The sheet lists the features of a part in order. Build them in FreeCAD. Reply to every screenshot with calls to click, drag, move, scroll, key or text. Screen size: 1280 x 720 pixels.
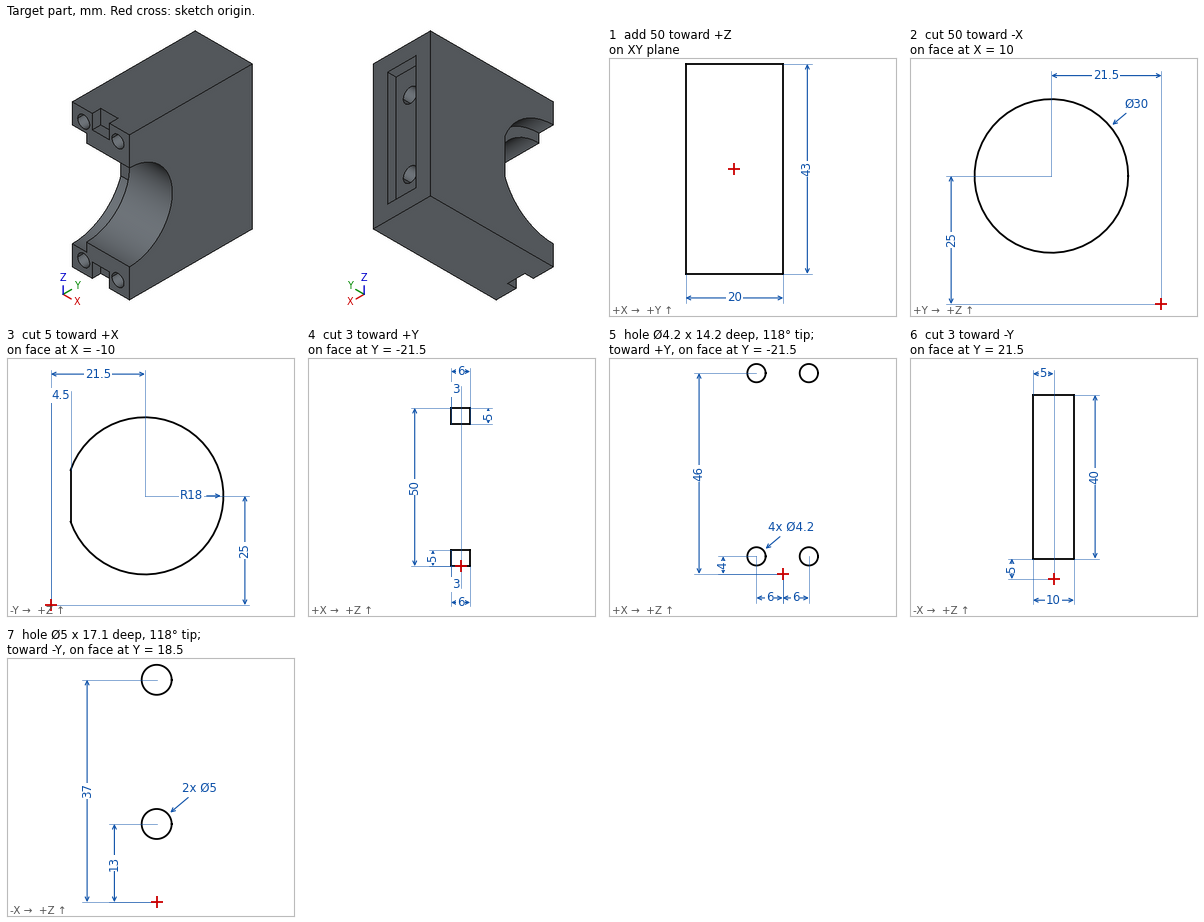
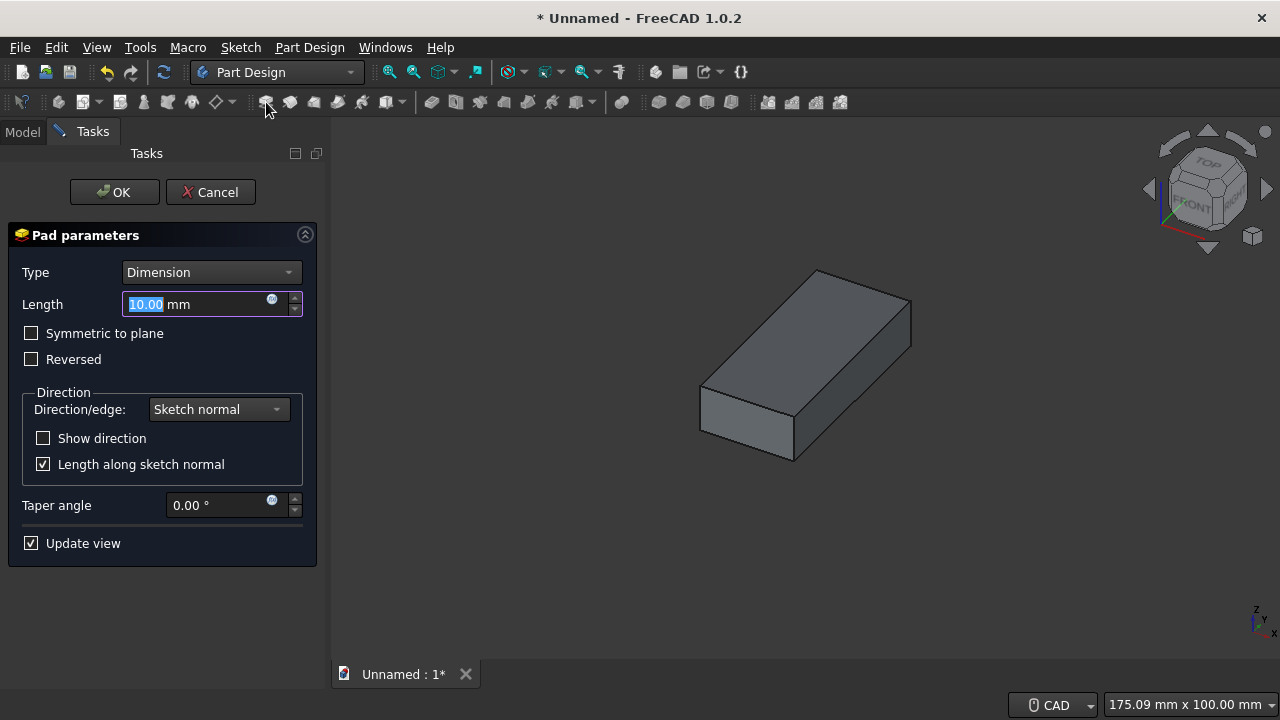
text(50)
key(Tab)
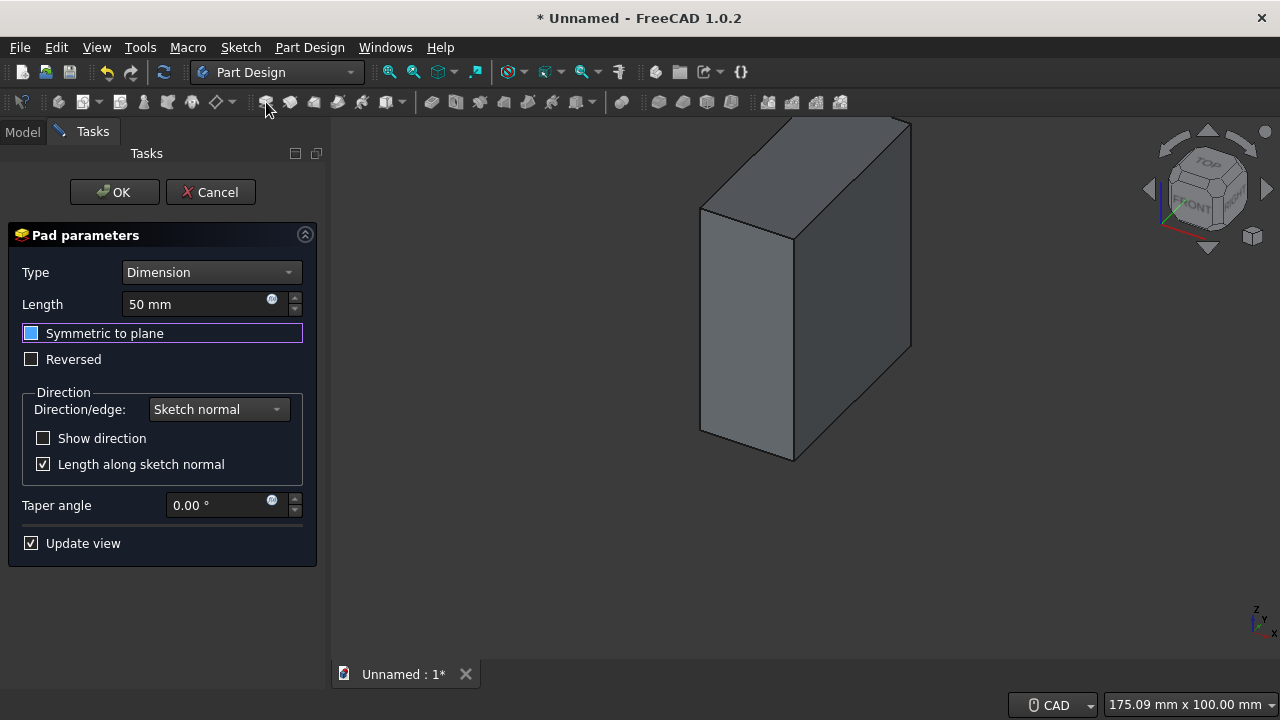
click(115, 192)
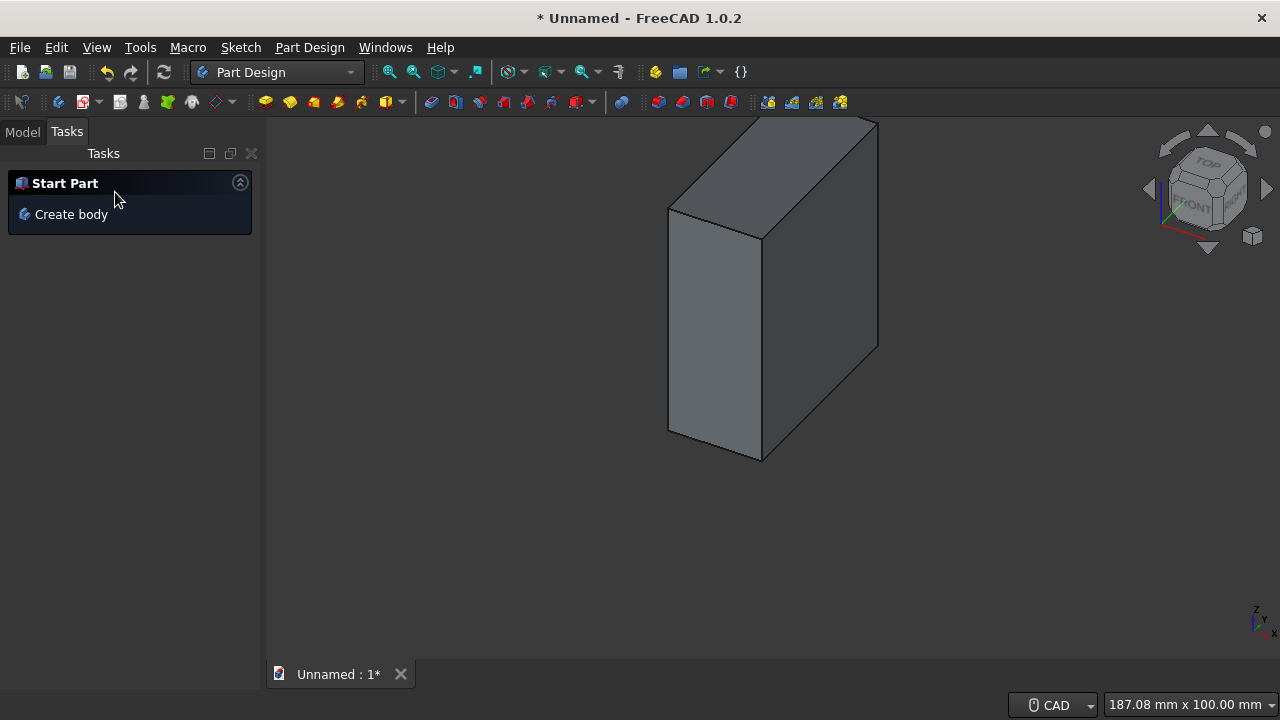
click(390, 72)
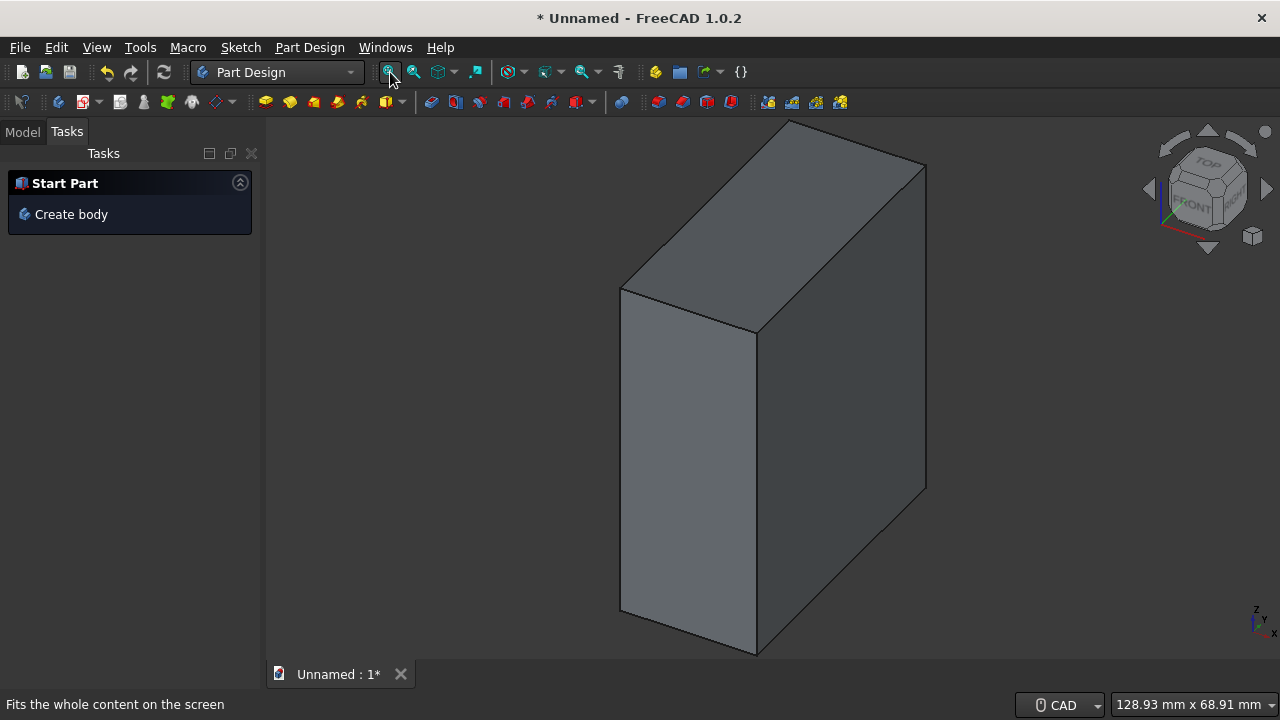
click(841, 410)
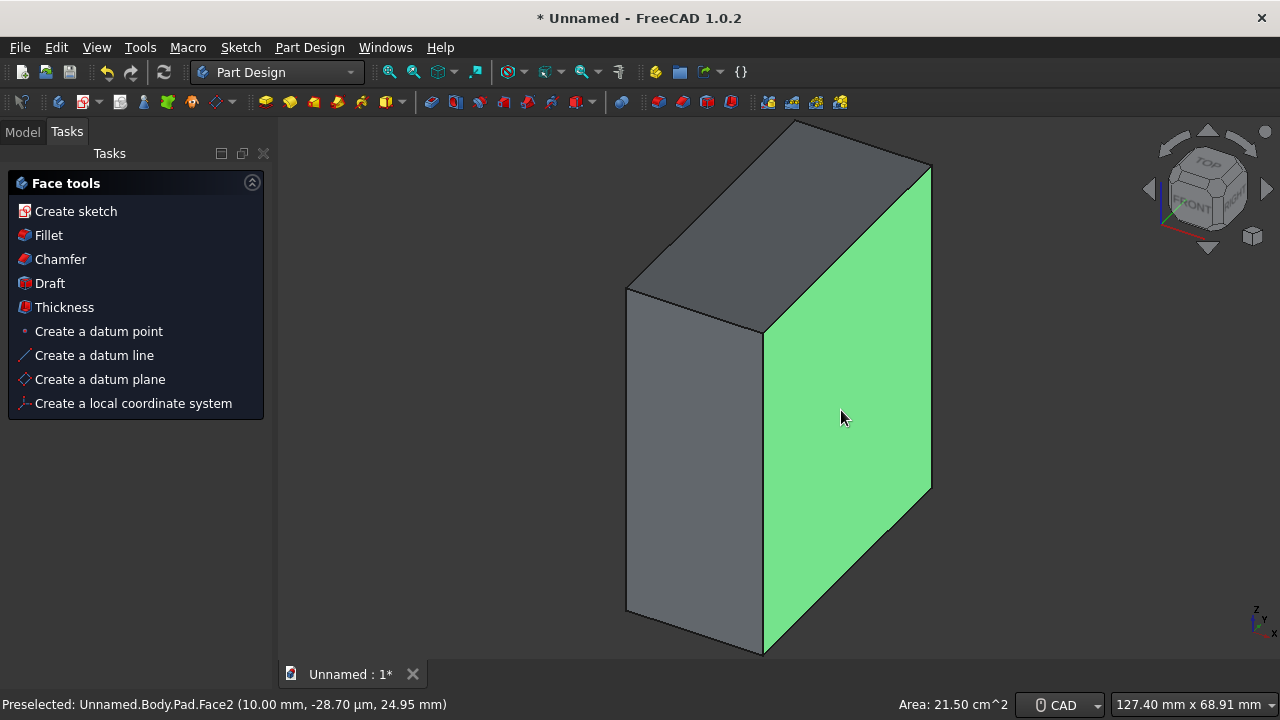
click(84, 102)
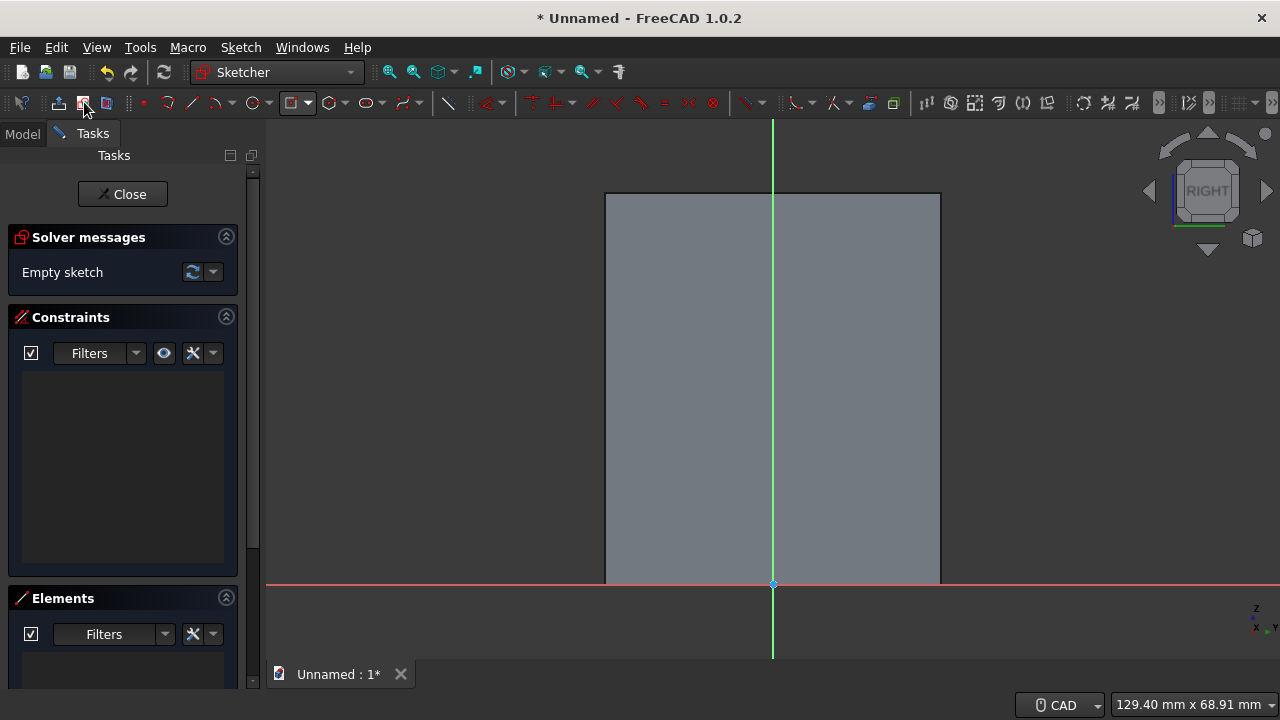
click(254, 104)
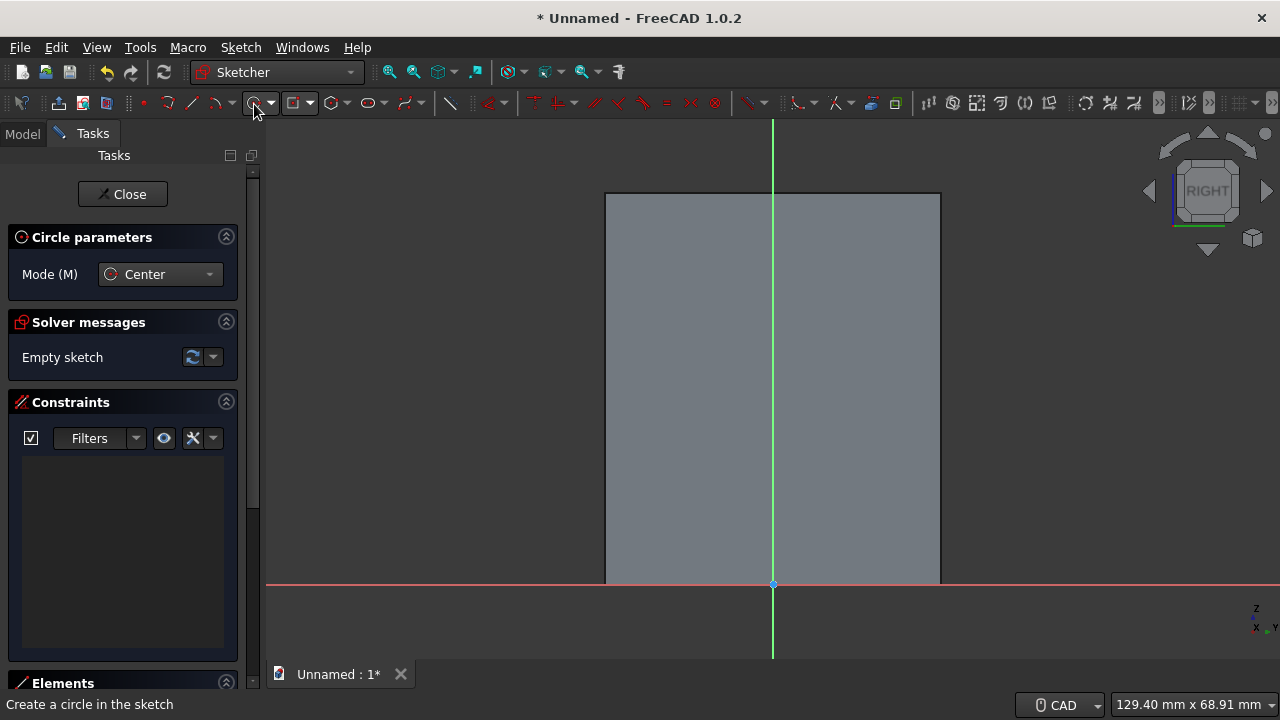
click(605, 389)
move(688, 306)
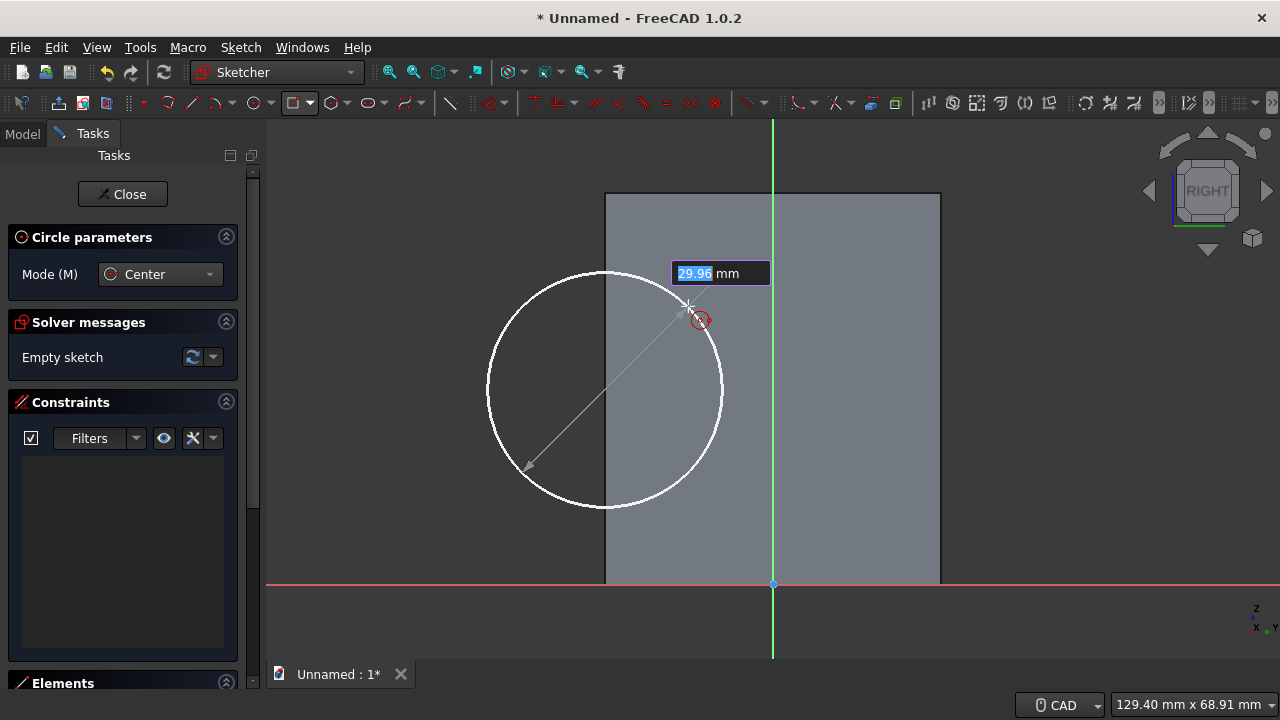
text(30)
key(Return)
key(Escape)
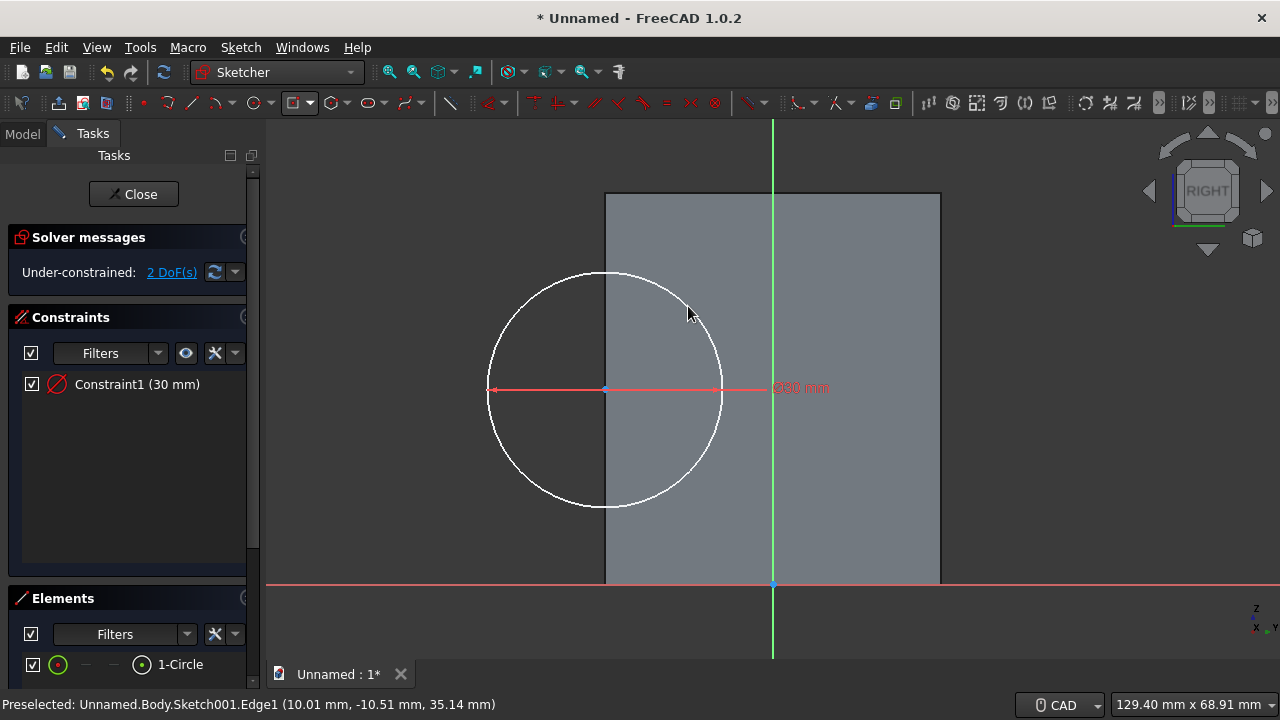
click(488, 104)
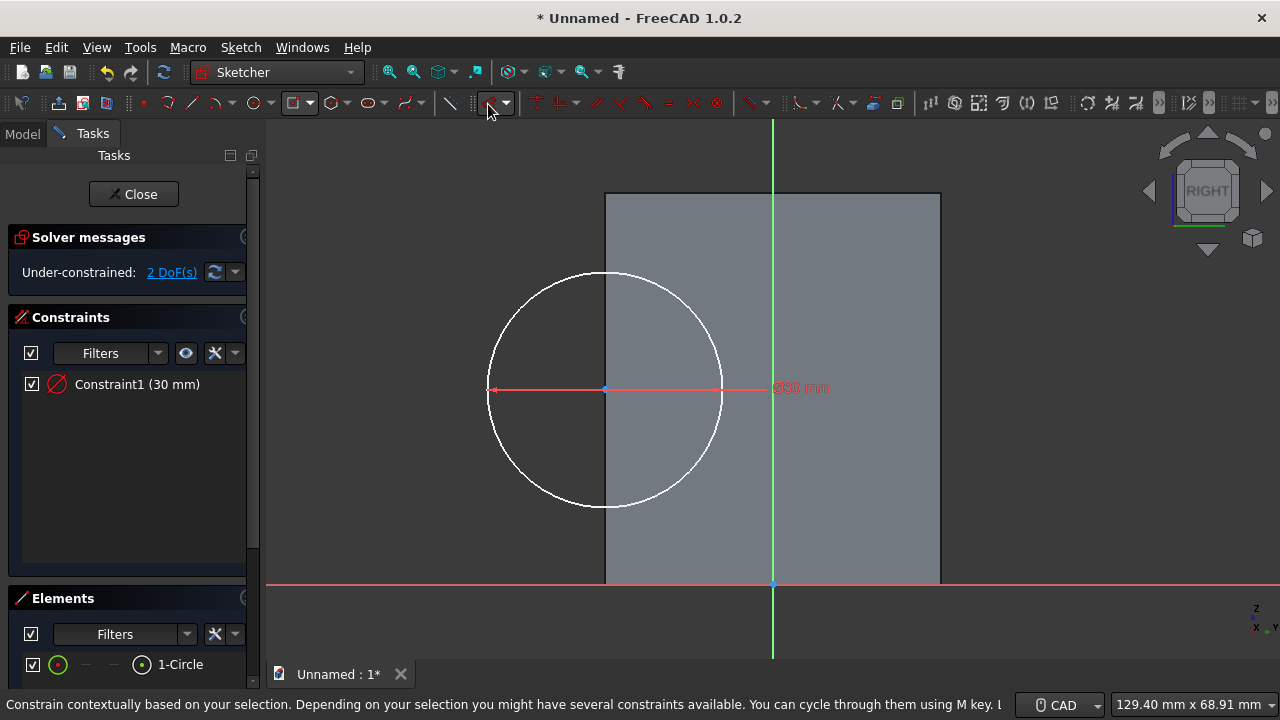
click(605, 390)
click(807, 487)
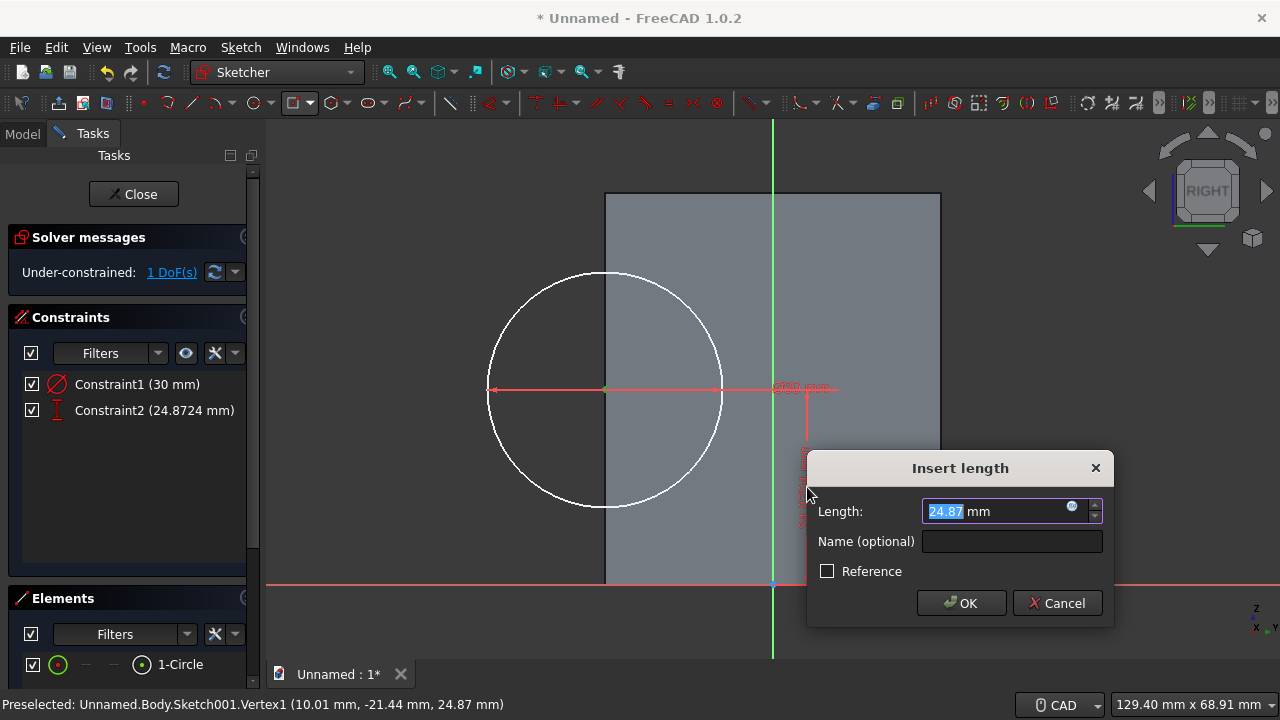
text(25)
key(Return)